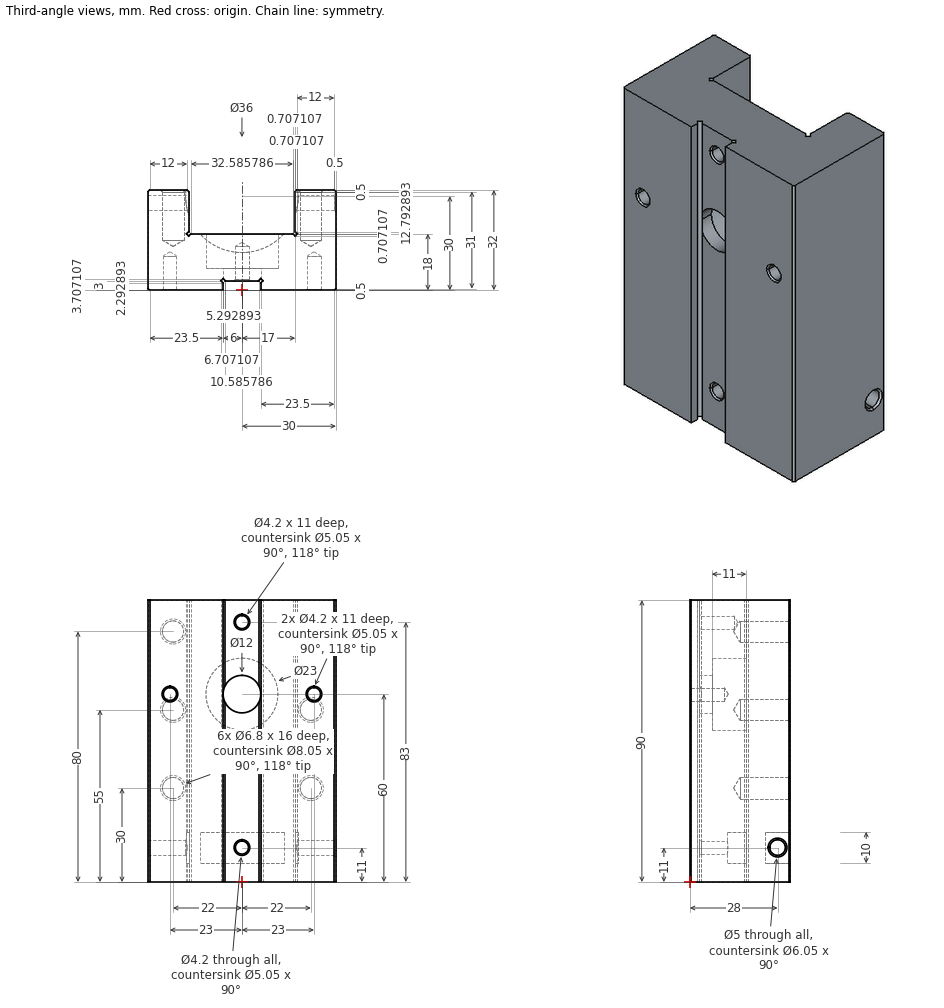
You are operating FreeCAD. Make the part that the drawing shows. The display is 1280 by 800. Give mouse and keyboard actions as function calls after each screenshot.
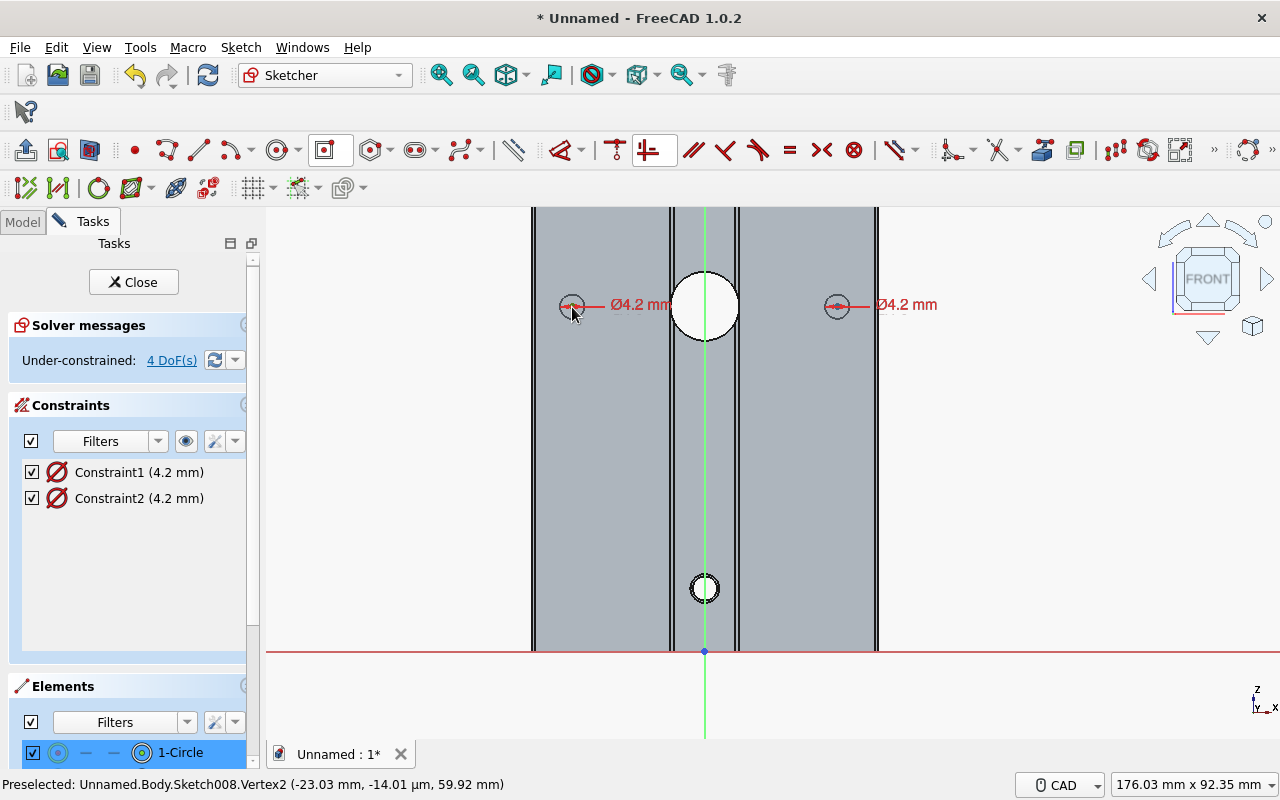
click(672, 150)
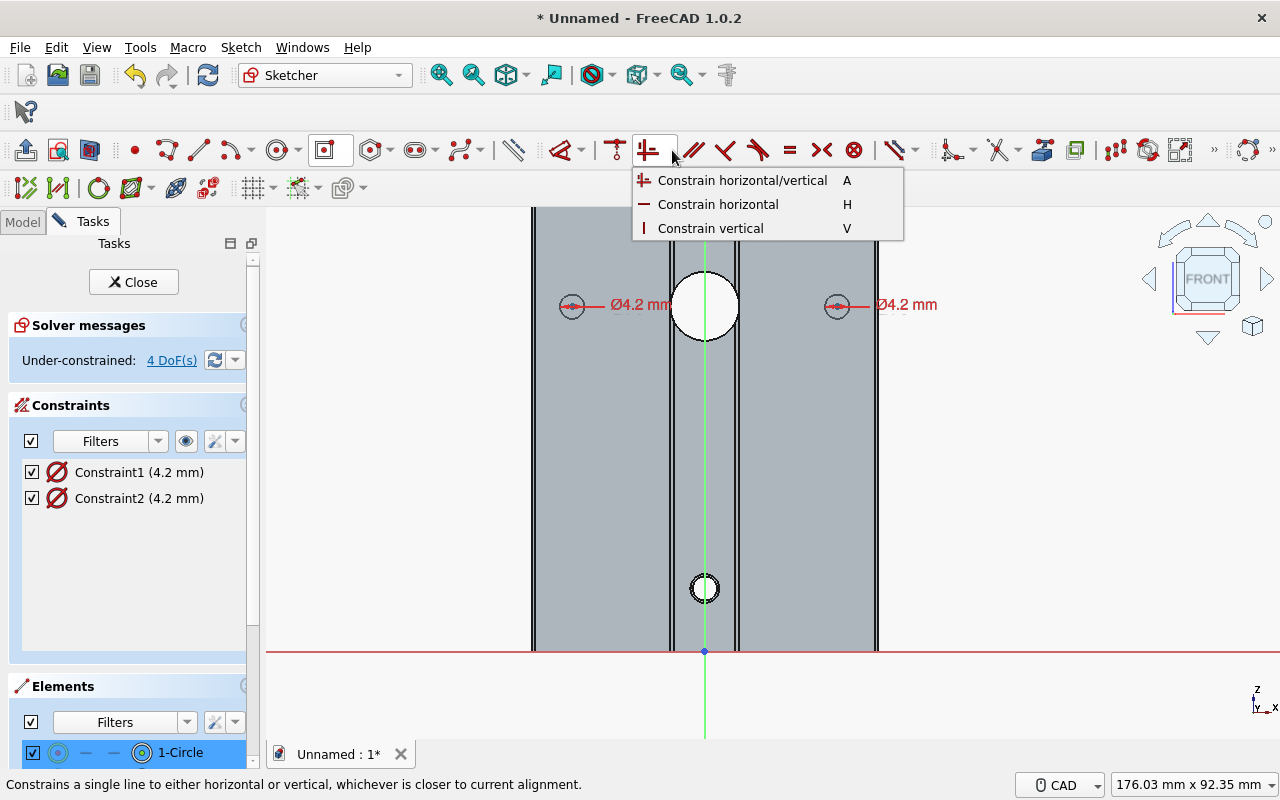
click(768, 204)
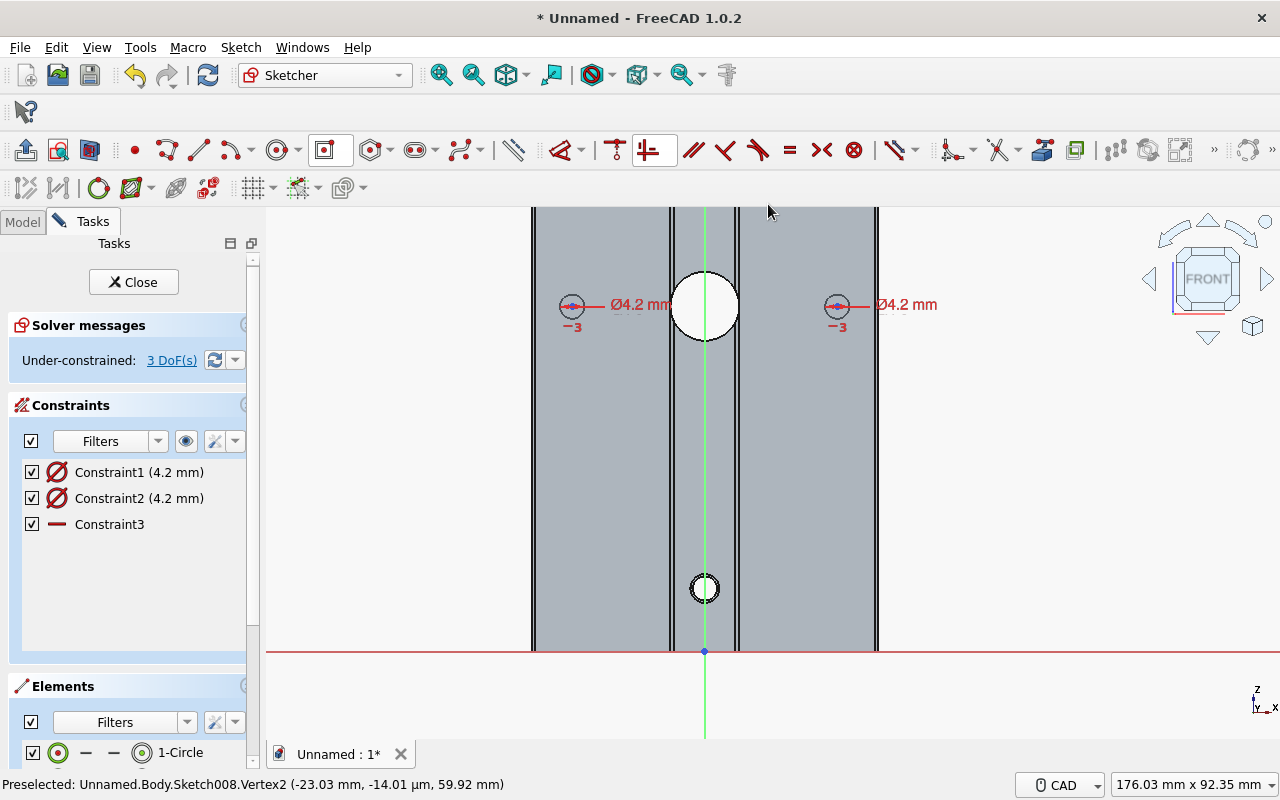
click(560, 150)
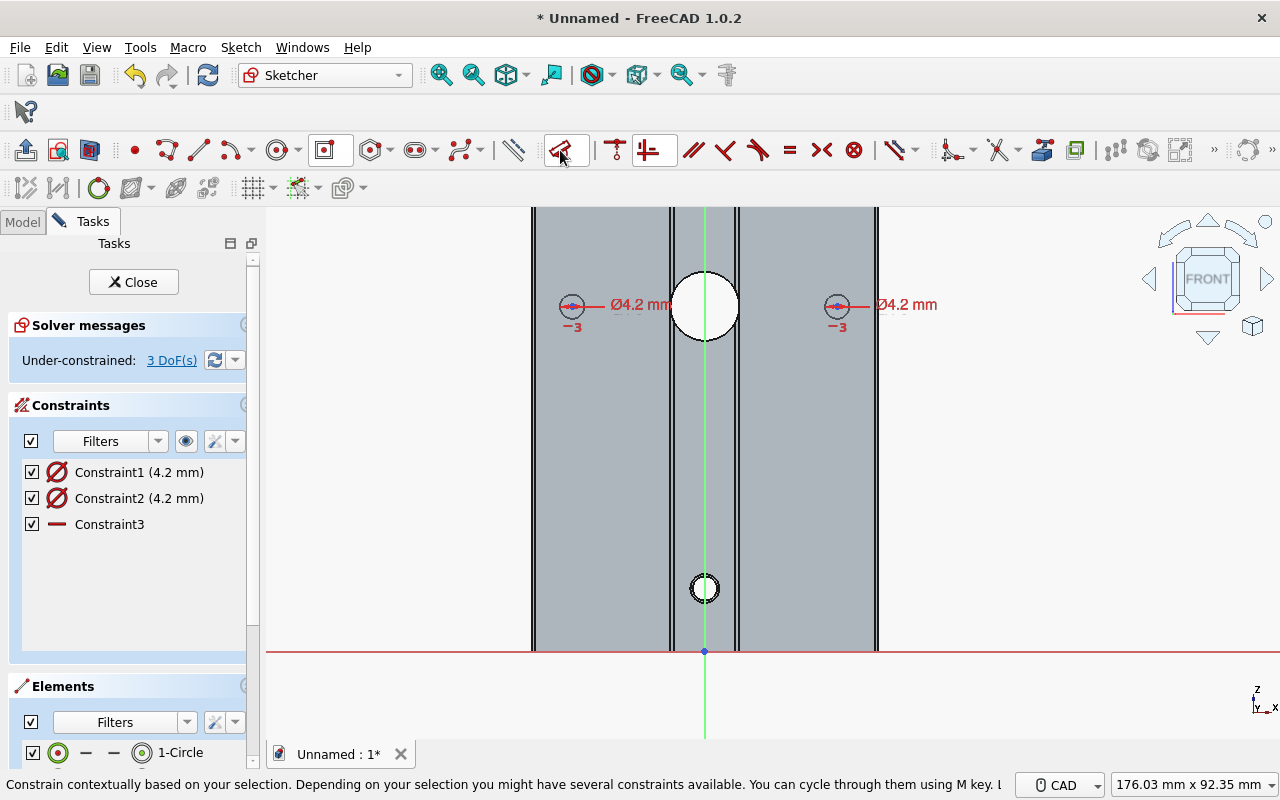
click(837, 307)
click(771, 686)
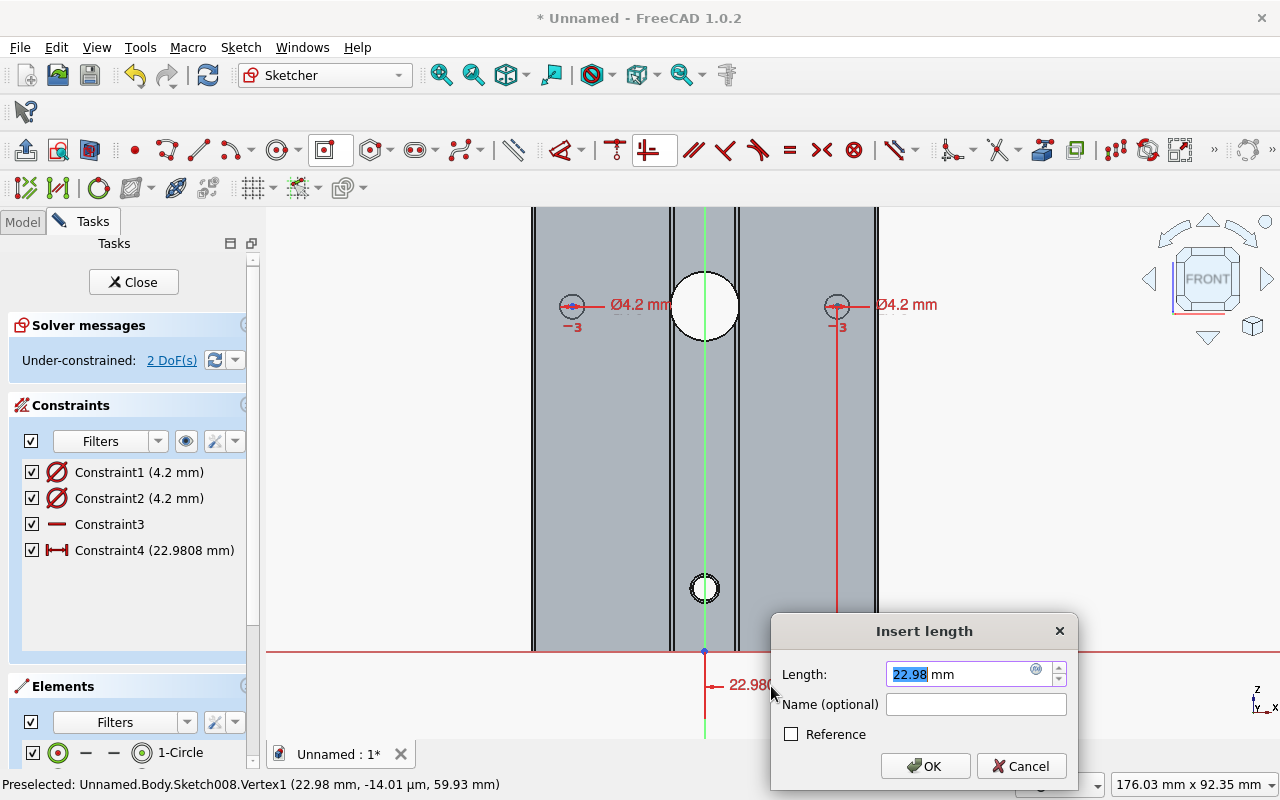
text(23)
key(Return)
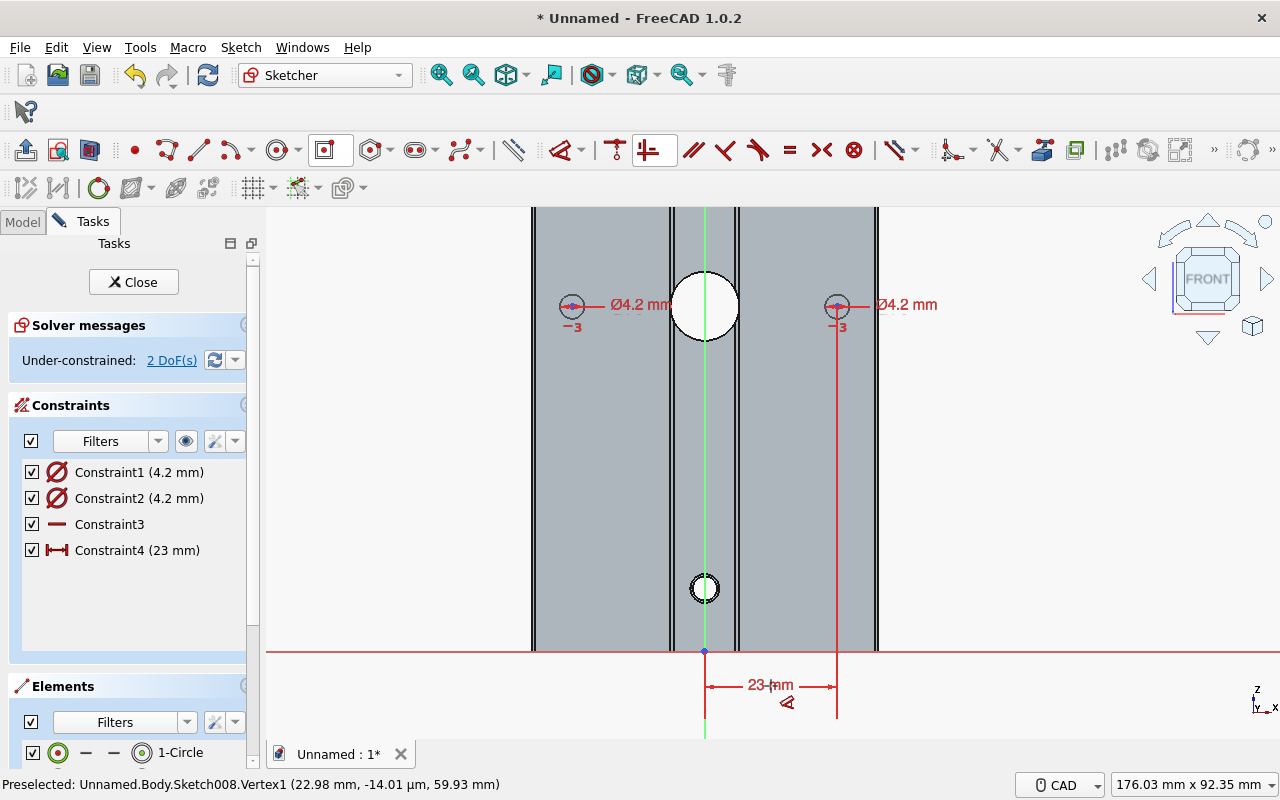
click(837, 307)
click(871, 479)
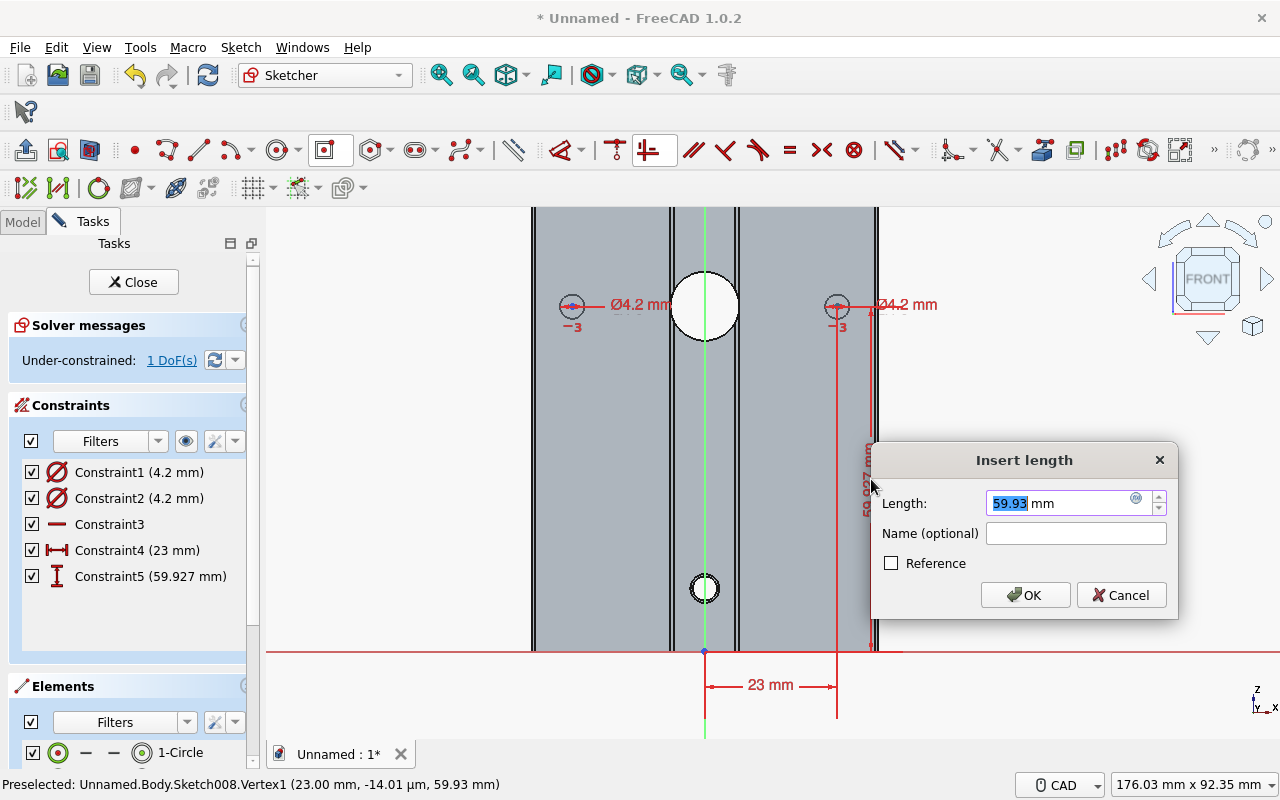
text(60)
key(Return)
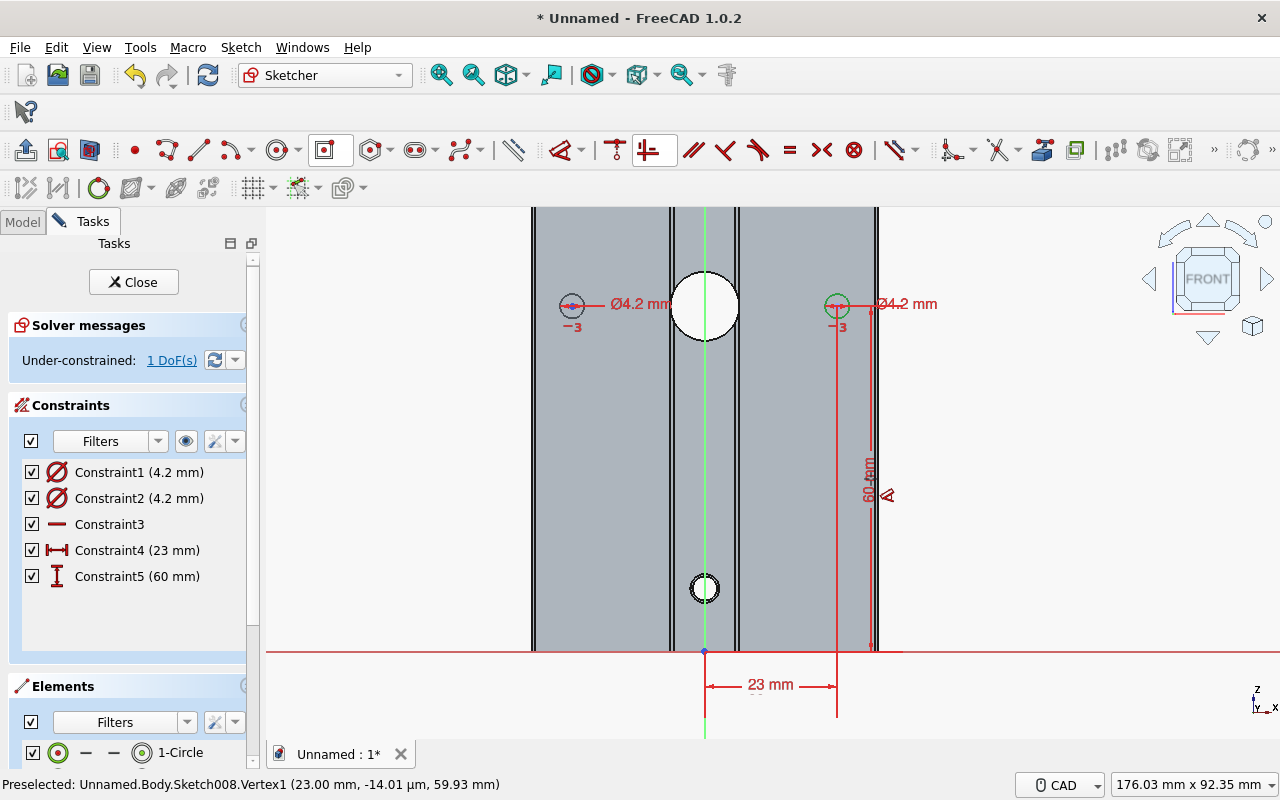
click(572, 306)
click(639, 686)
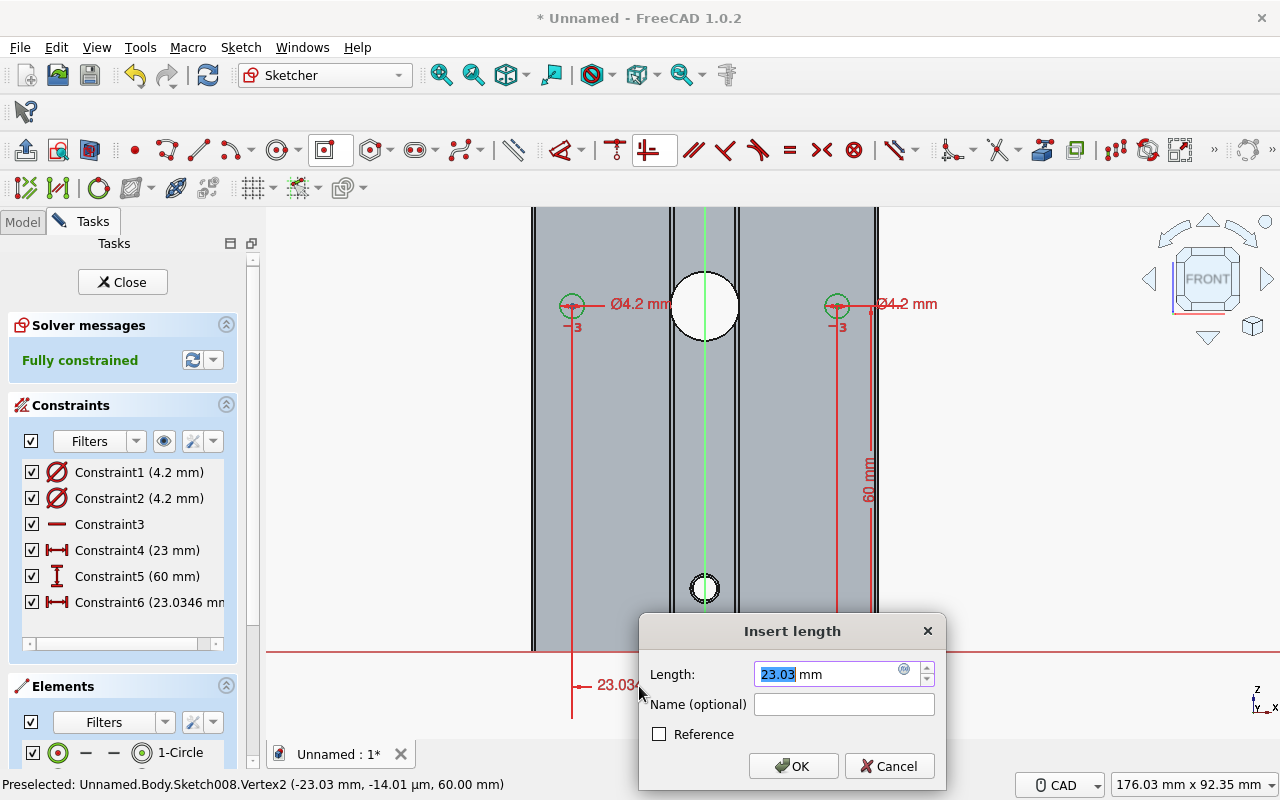
text(23)
key(Return)
key(Escape)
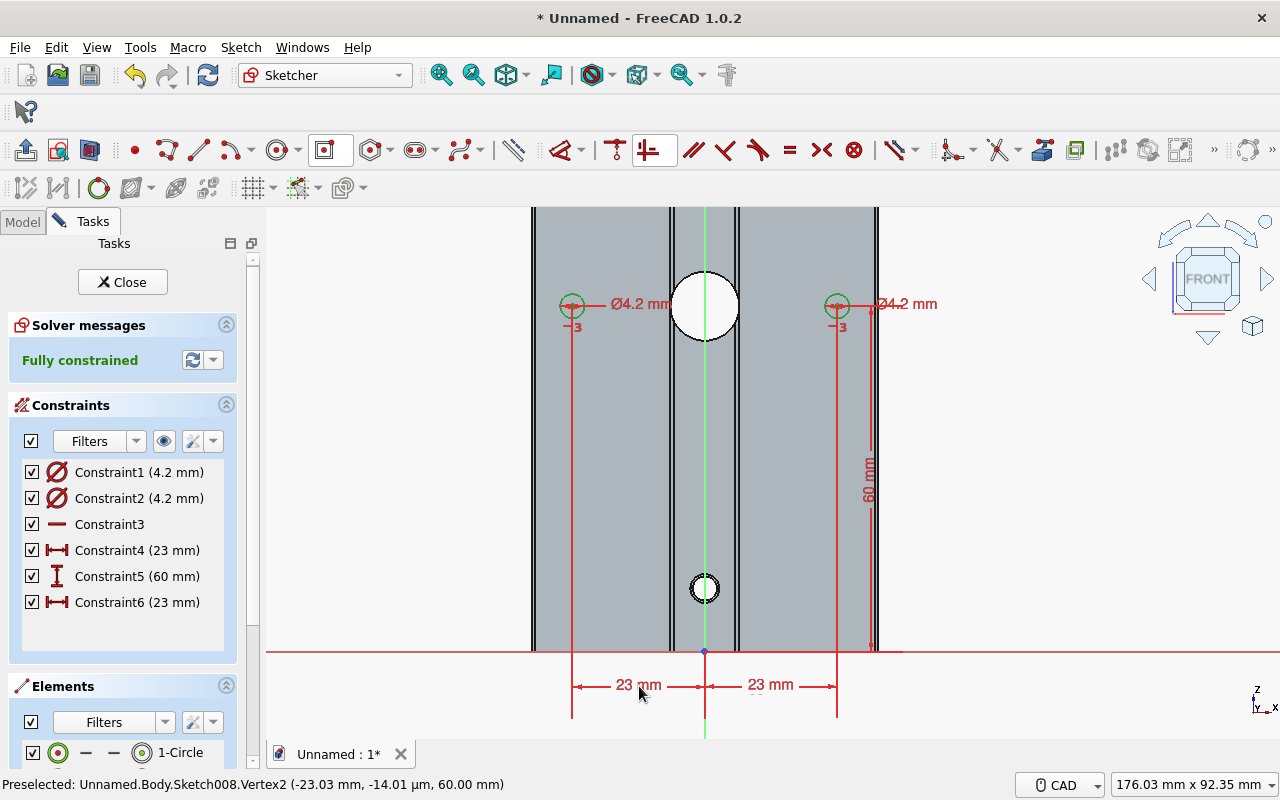
click(123, 282)